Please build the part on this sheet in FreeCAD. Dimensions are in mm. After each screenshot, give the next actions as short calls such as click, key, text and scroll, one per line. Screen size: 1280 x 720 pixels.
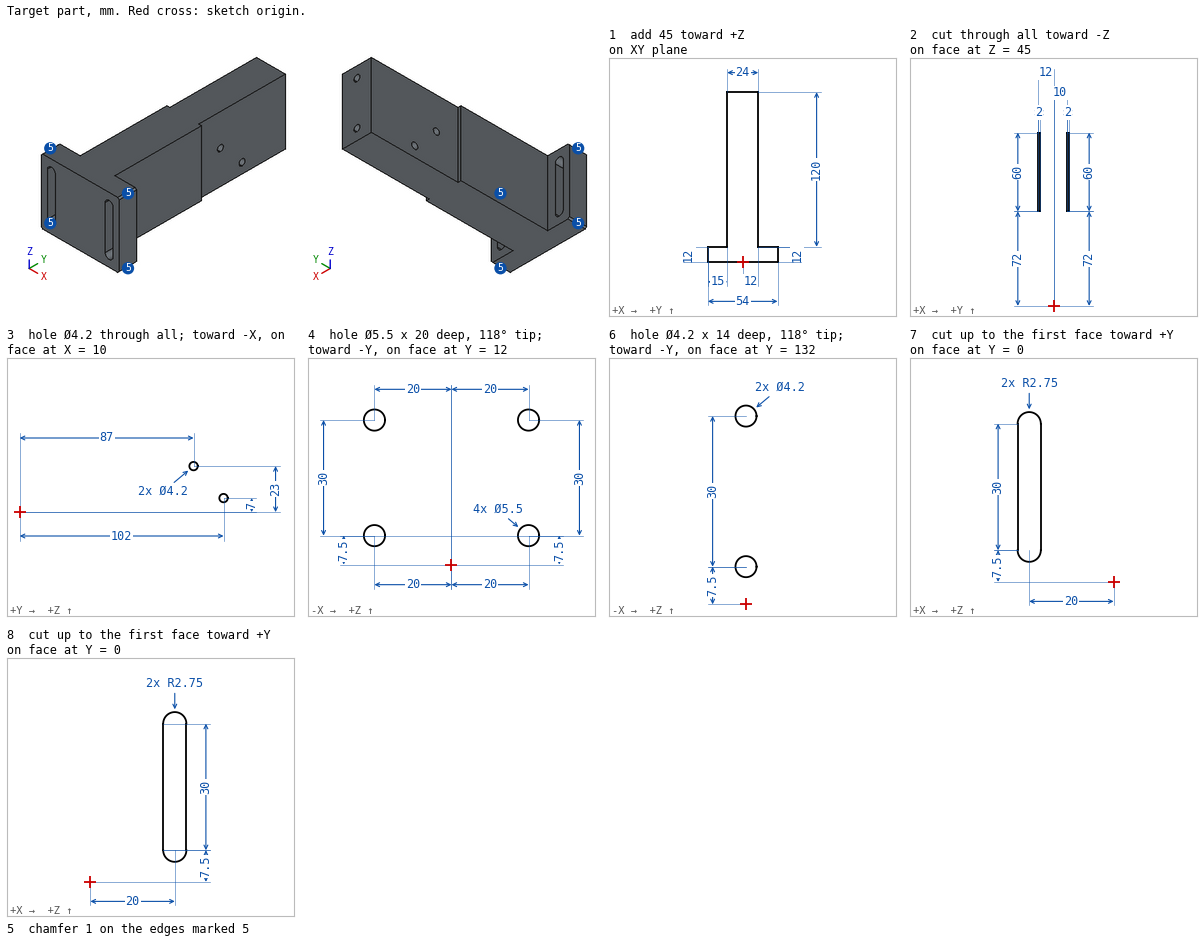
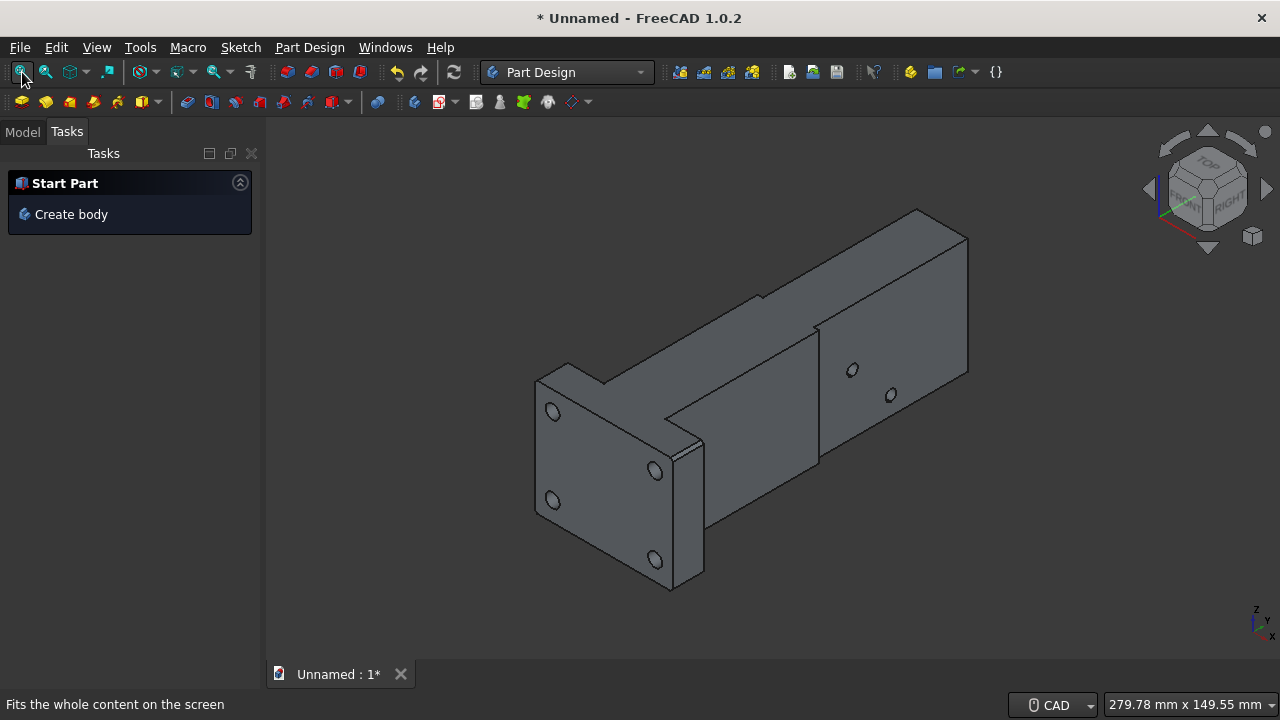
click(604, 485)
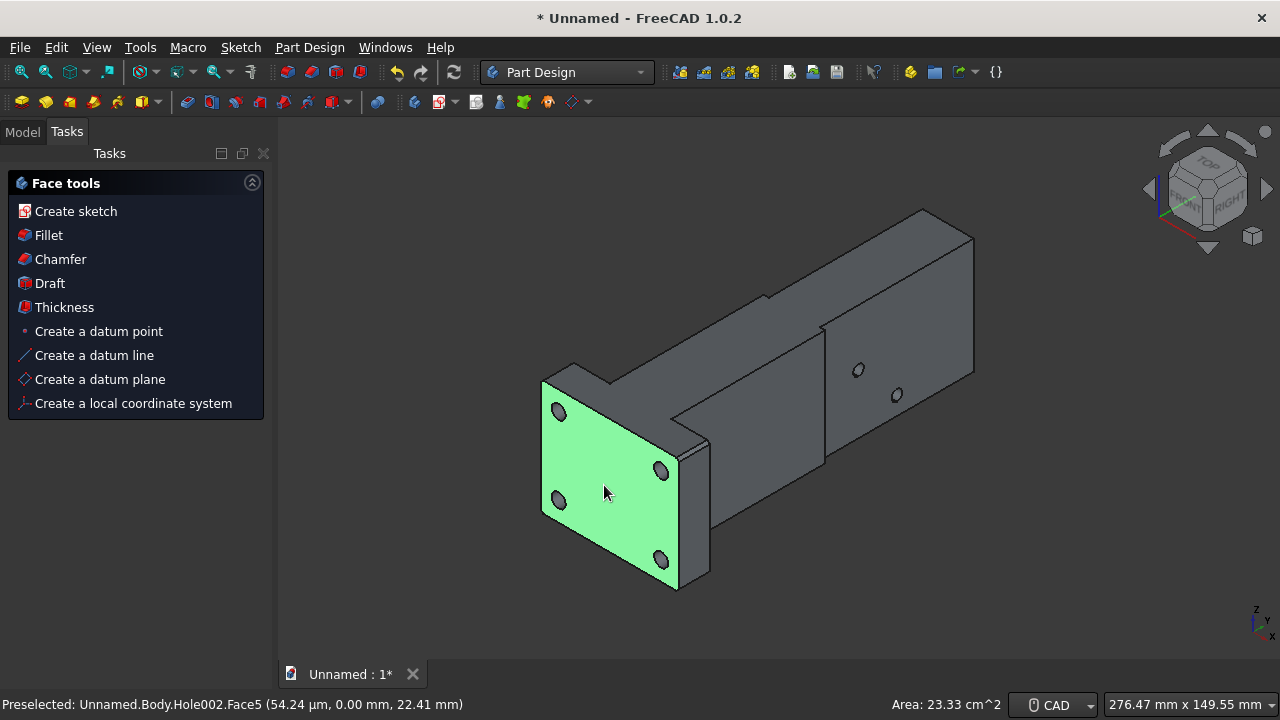
click(440, 102)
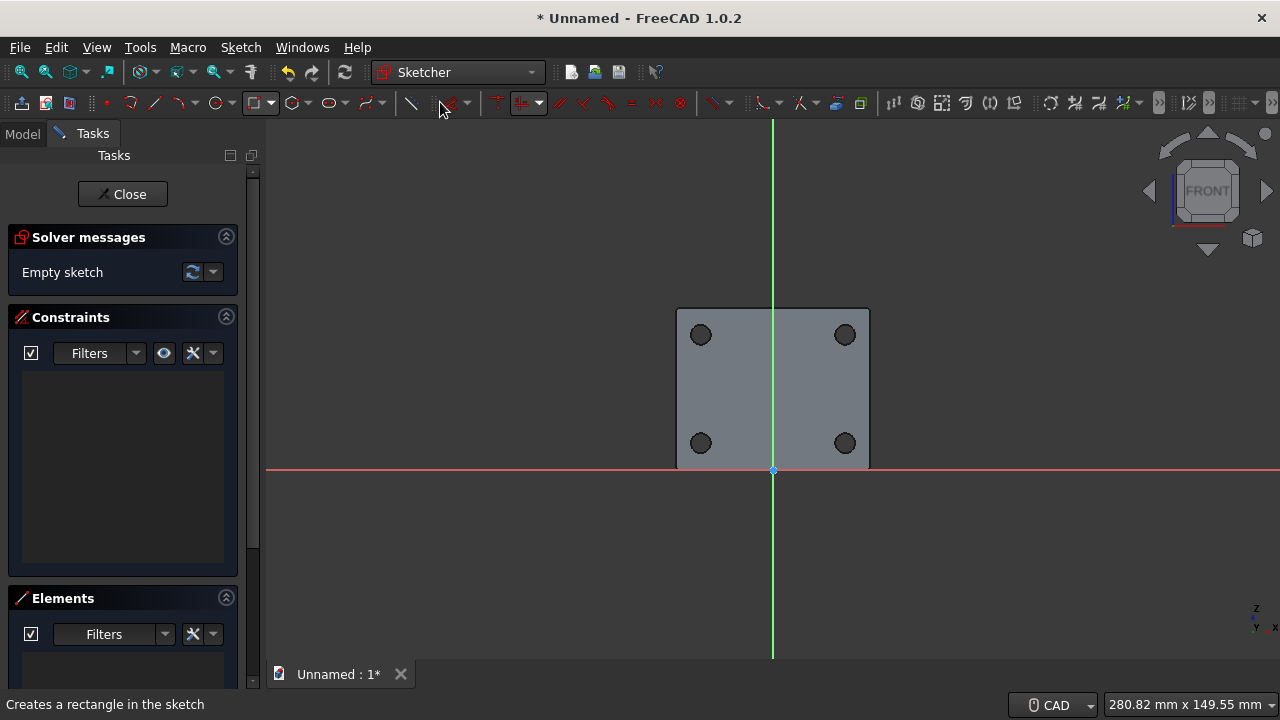
scroll(754, 405, up, 4)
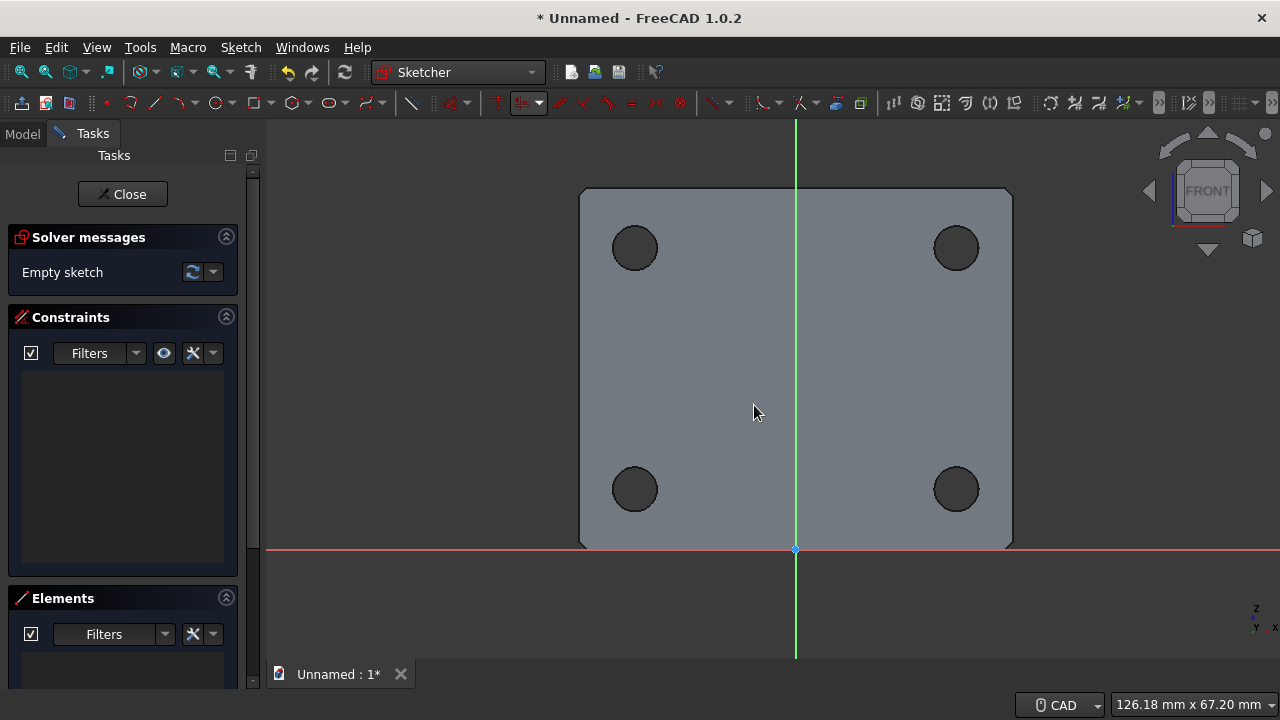
click(330, 104)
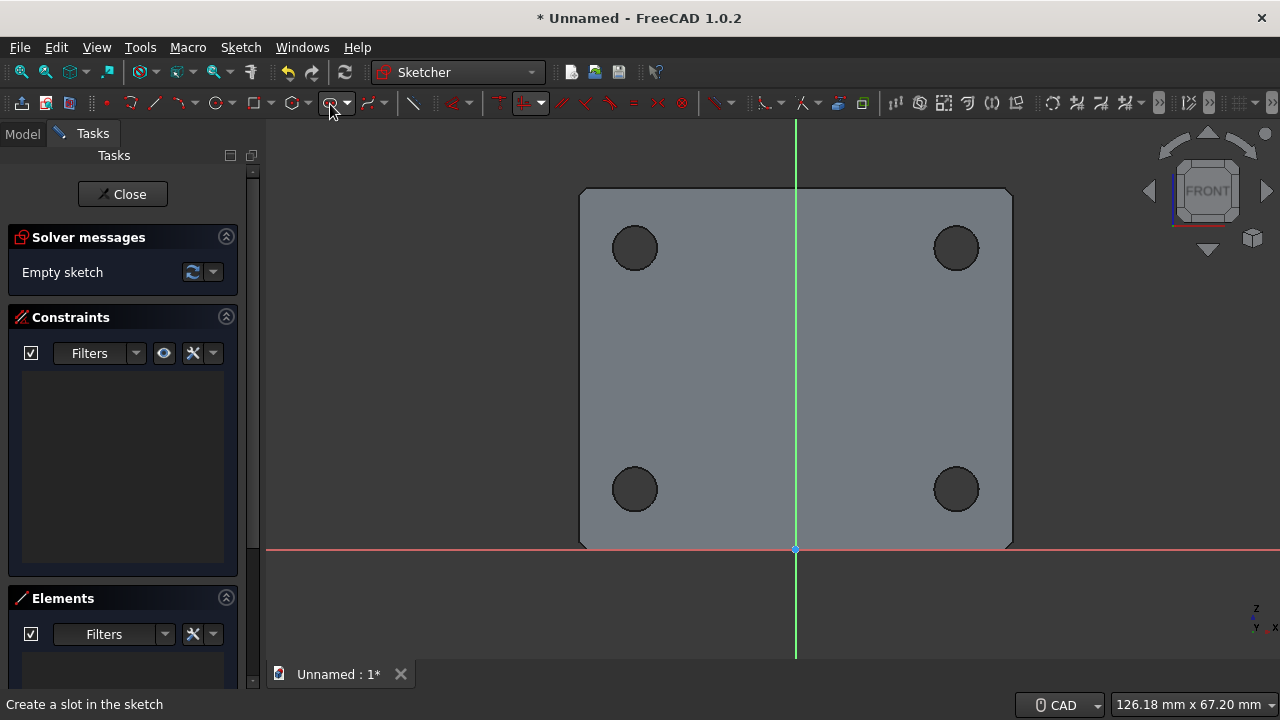
click(635, 489)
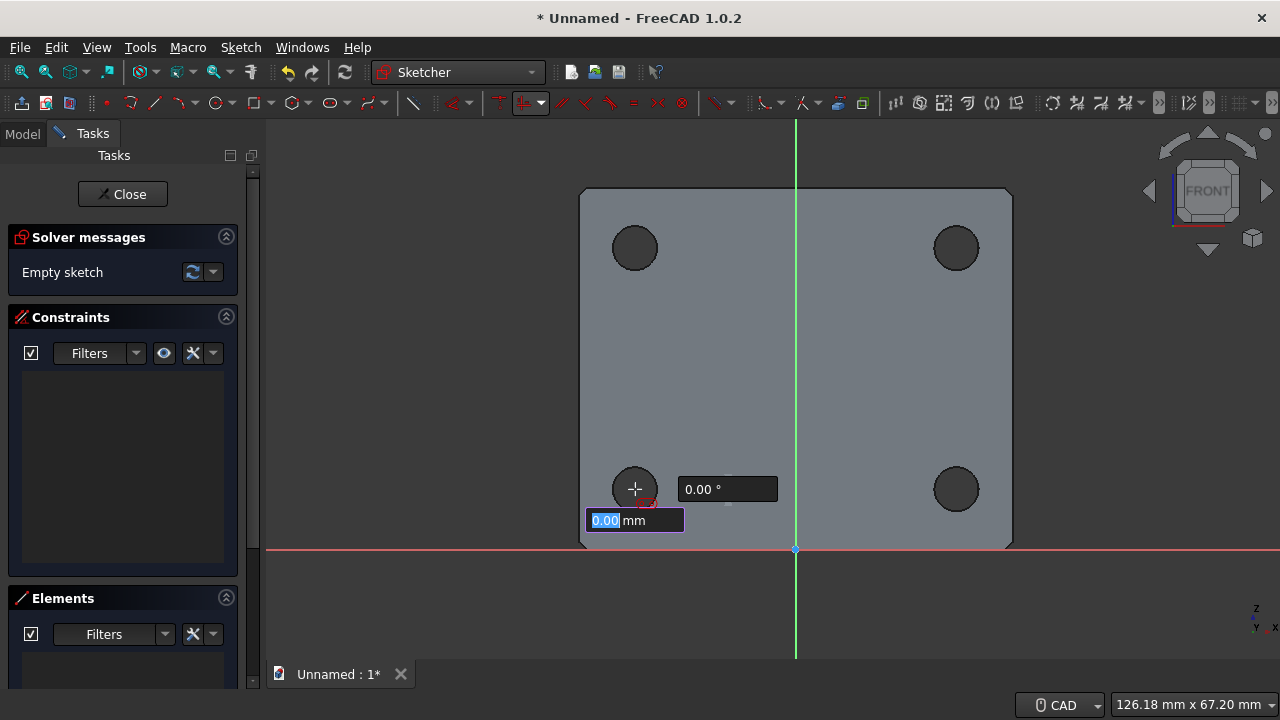
click(635, 248)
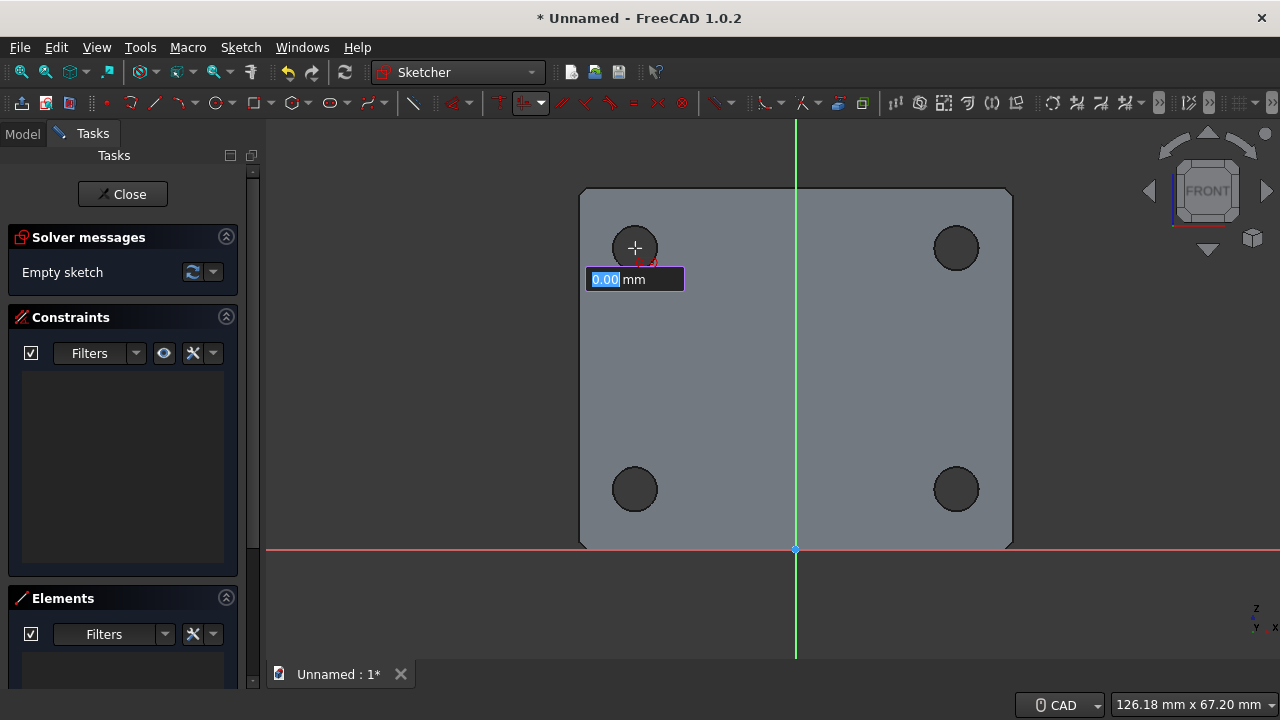
click(657, 369)
key(Escape)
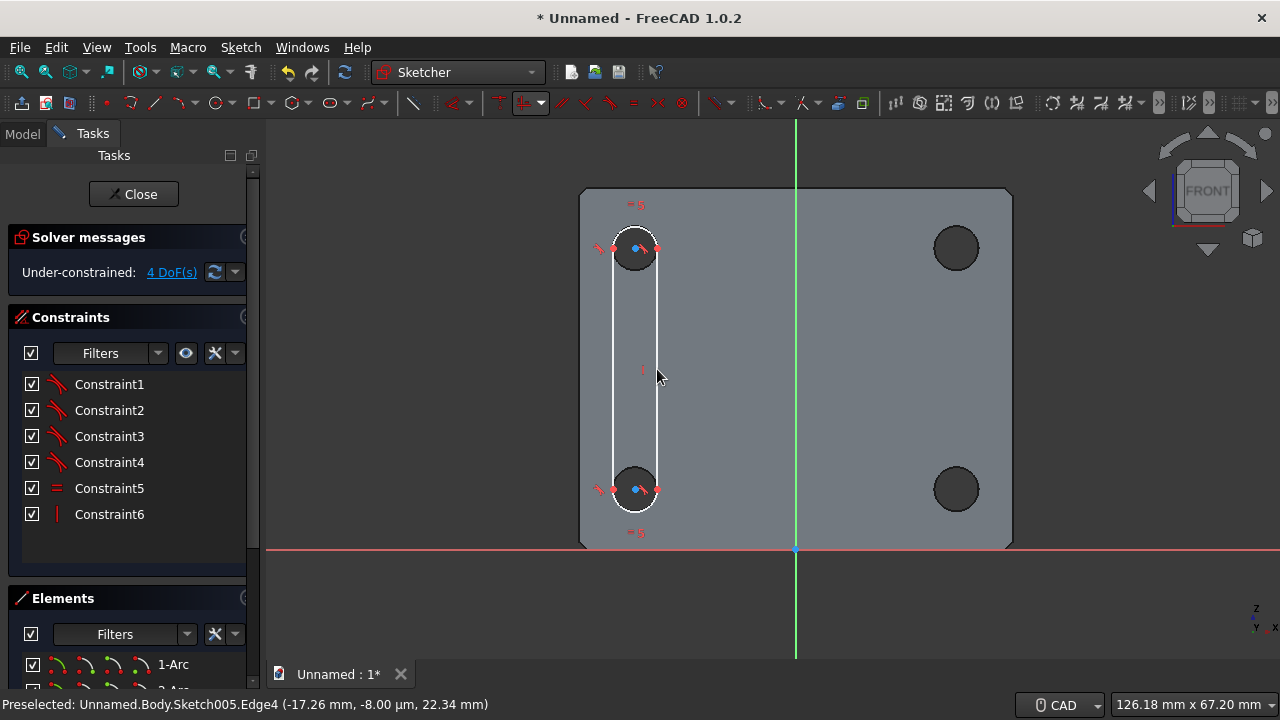
click(452, 104)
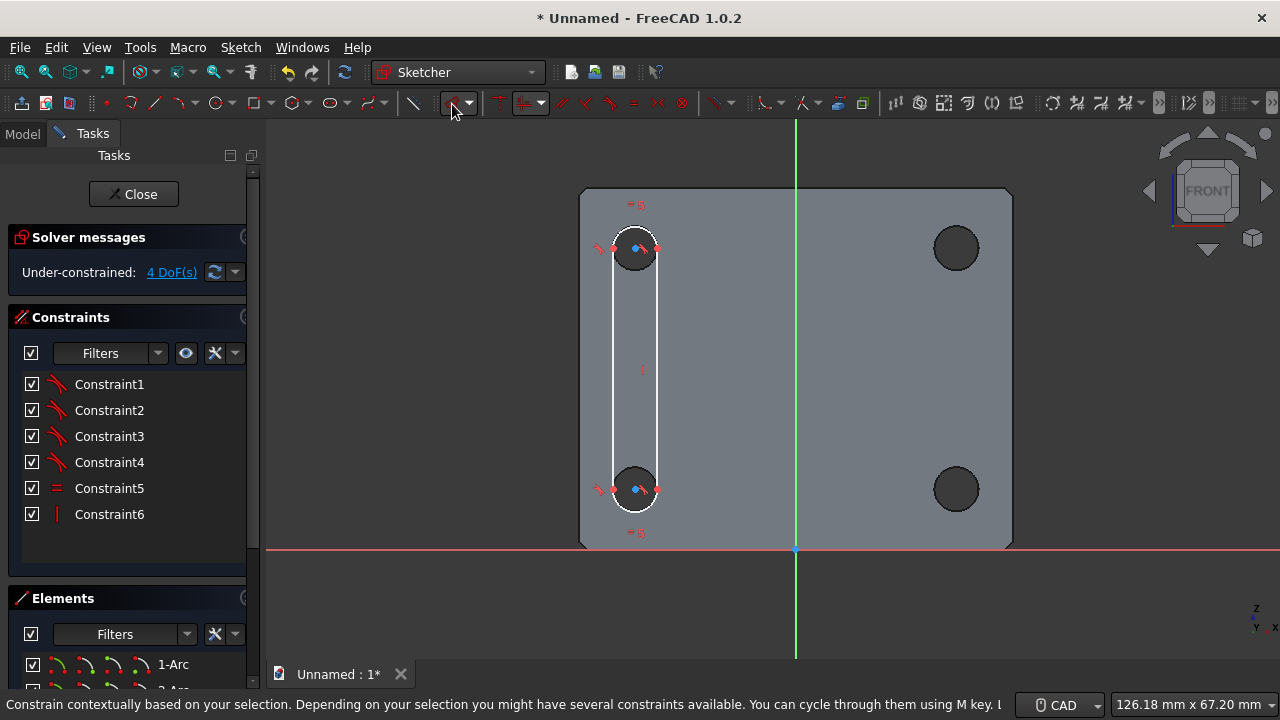
scroll(622, 508, up, 3)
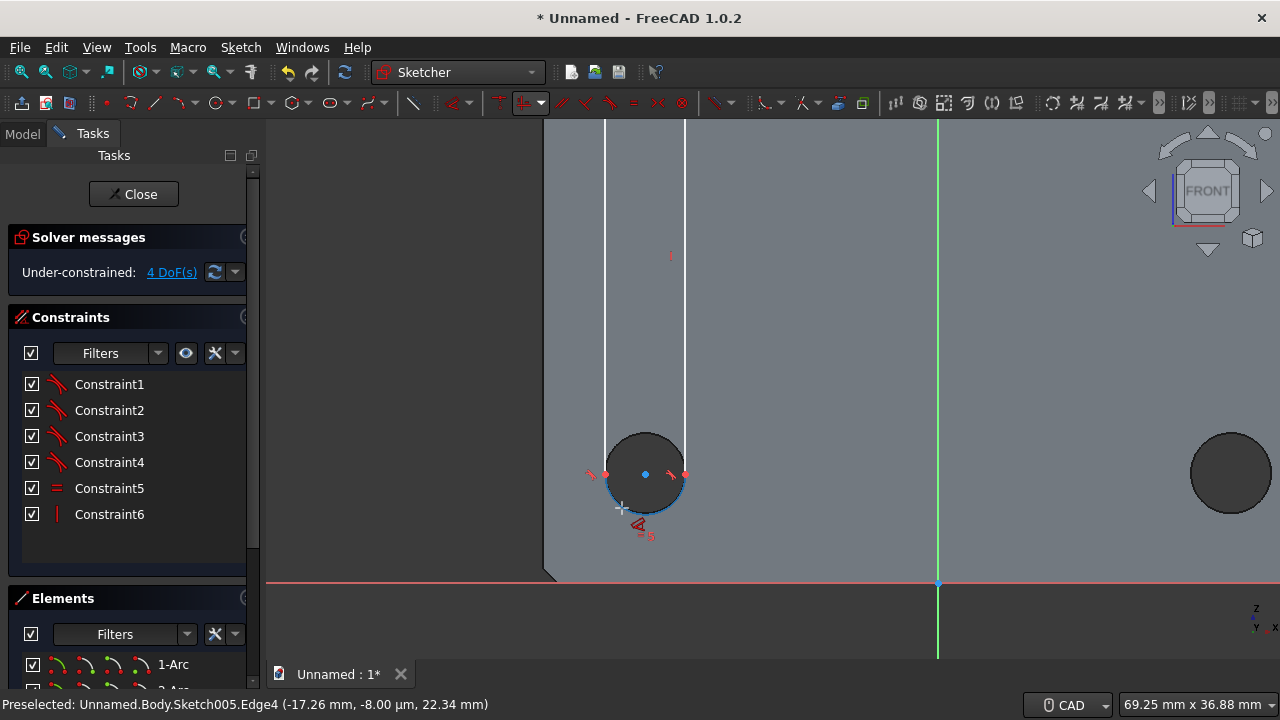
click(622, 507)
click(603, 533)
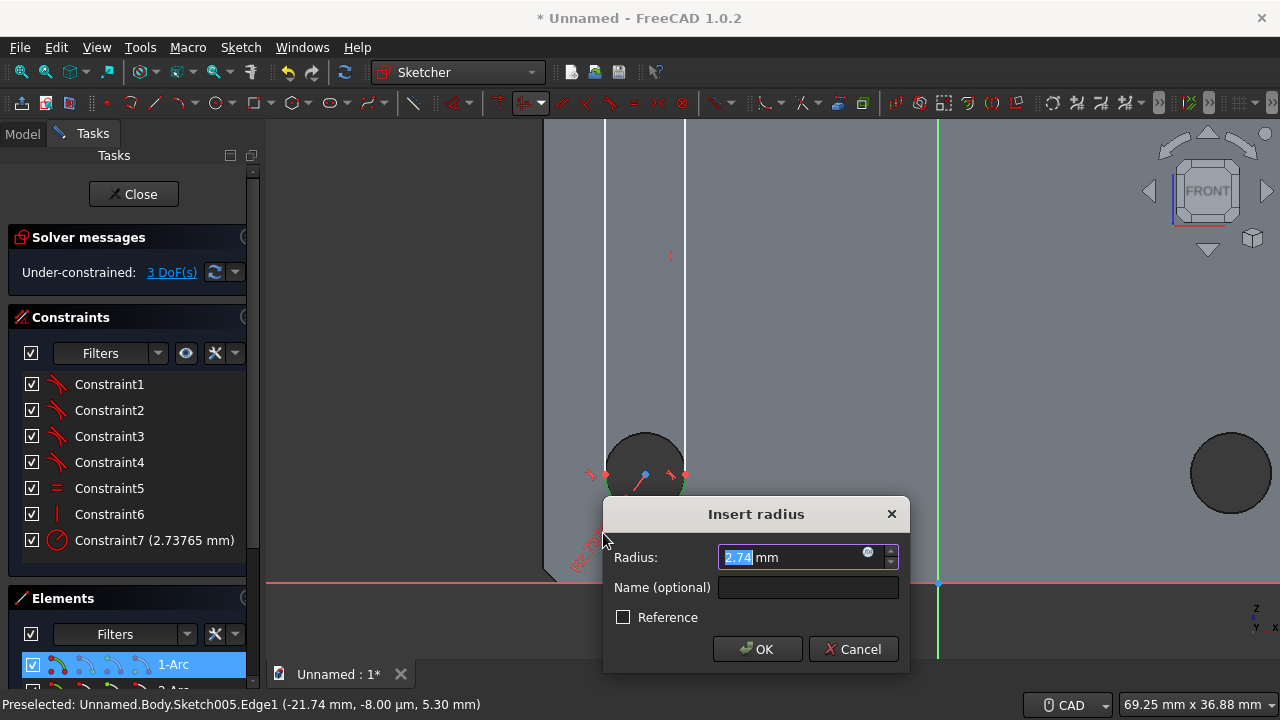
text(2.75)
key(Return)